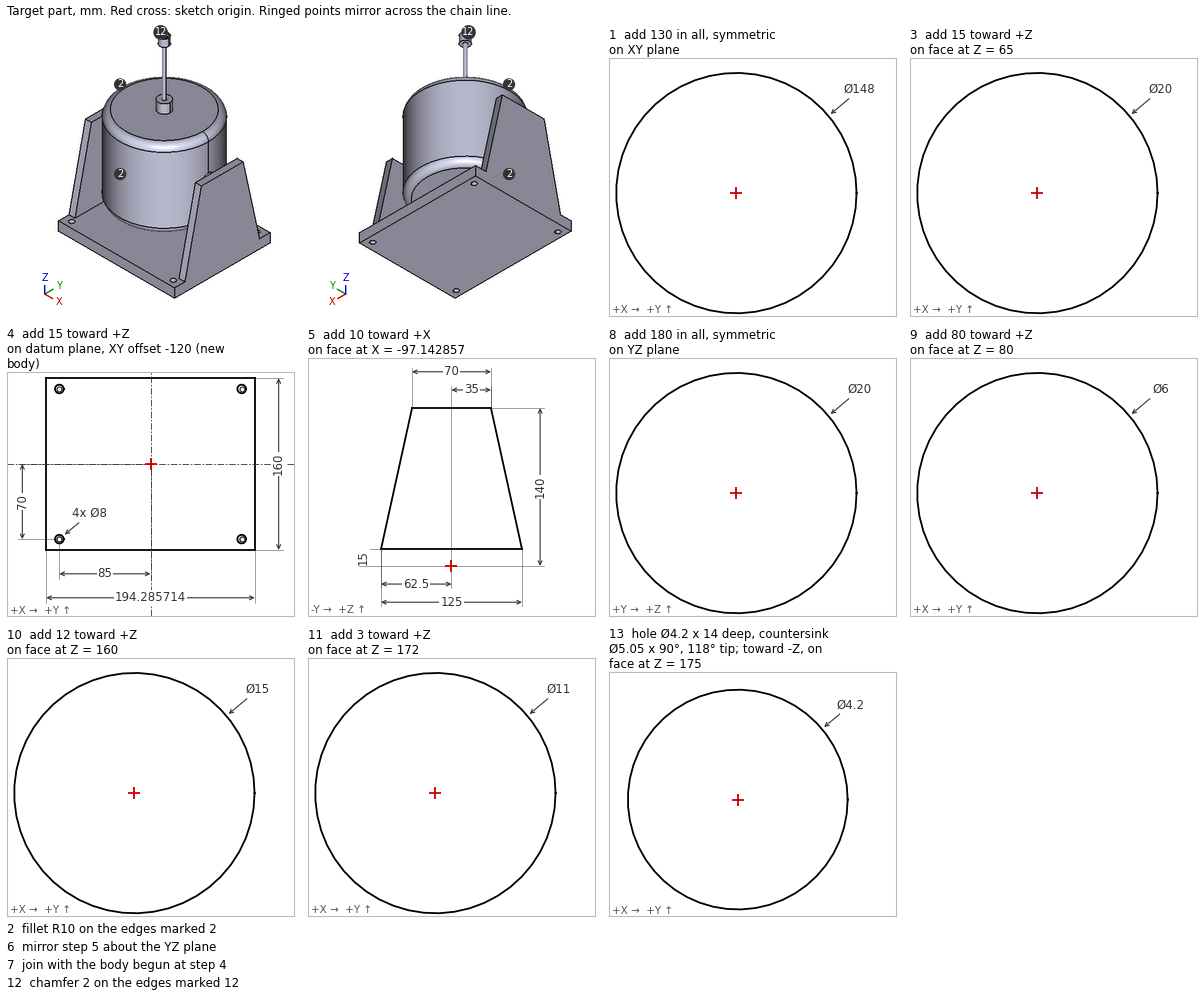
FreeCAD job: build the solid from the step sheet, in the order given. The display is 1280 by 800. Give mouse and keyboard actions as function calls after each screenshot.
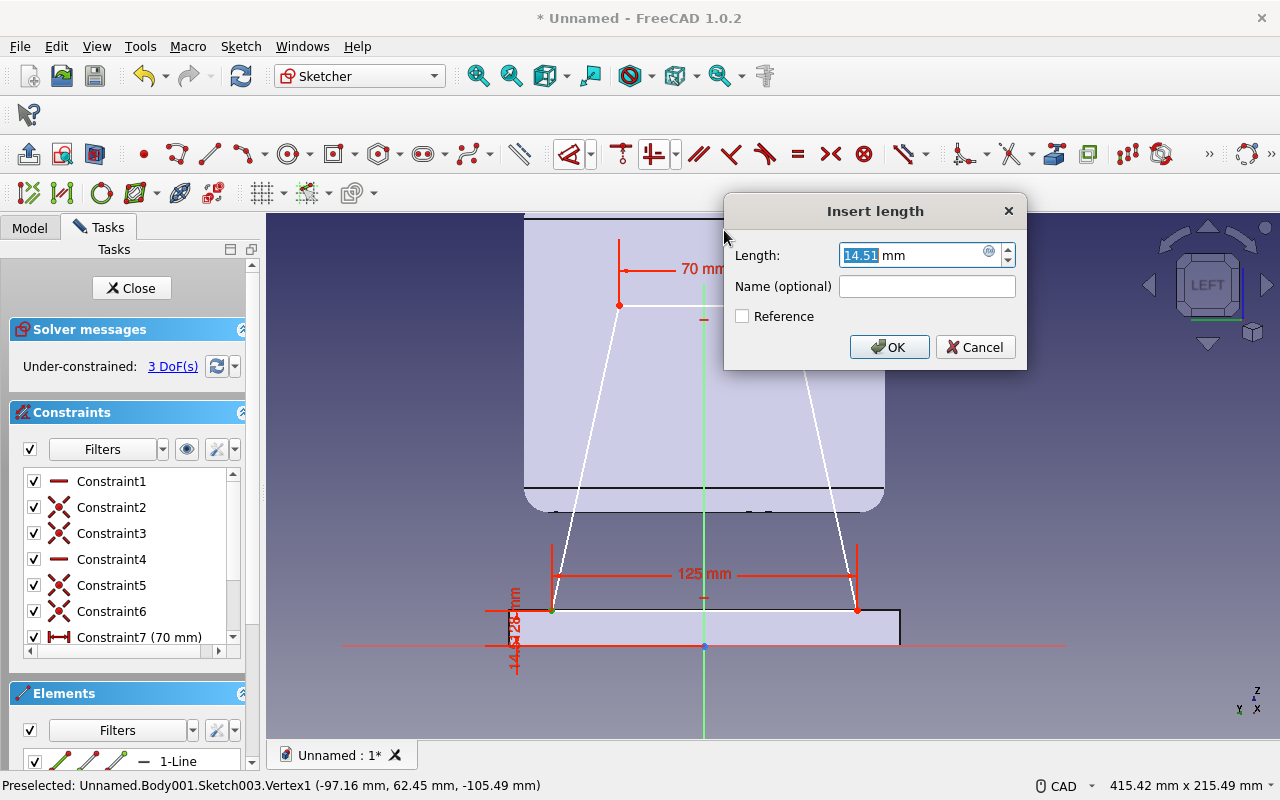
text(15)
key(Return)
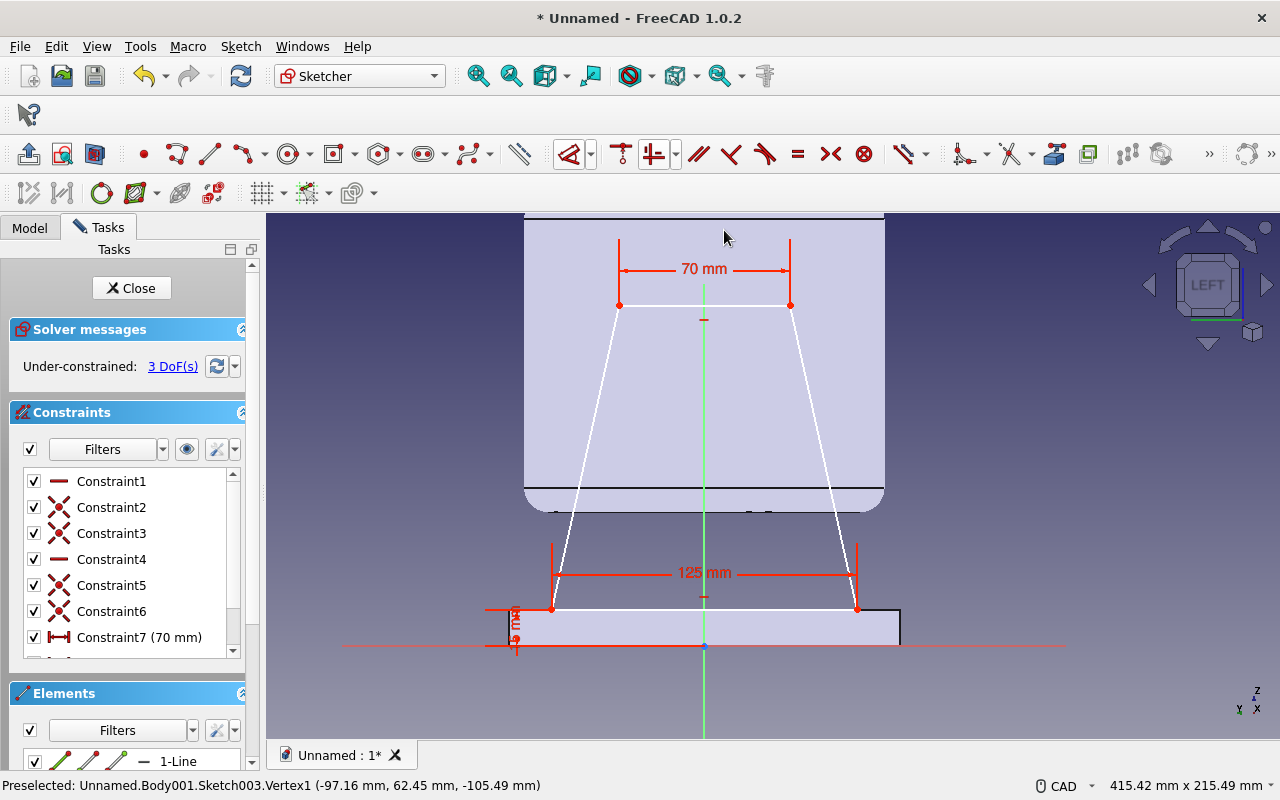
click(790, 306)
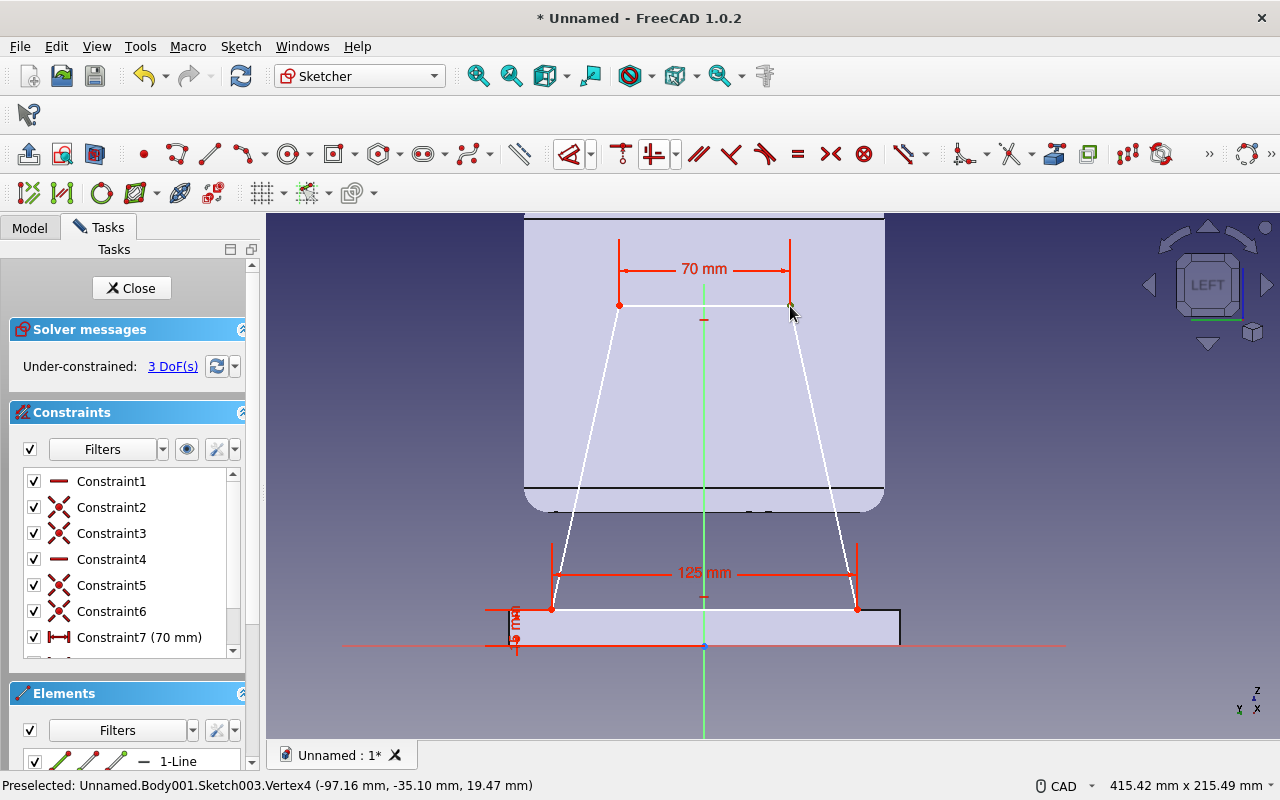
click(590, 154)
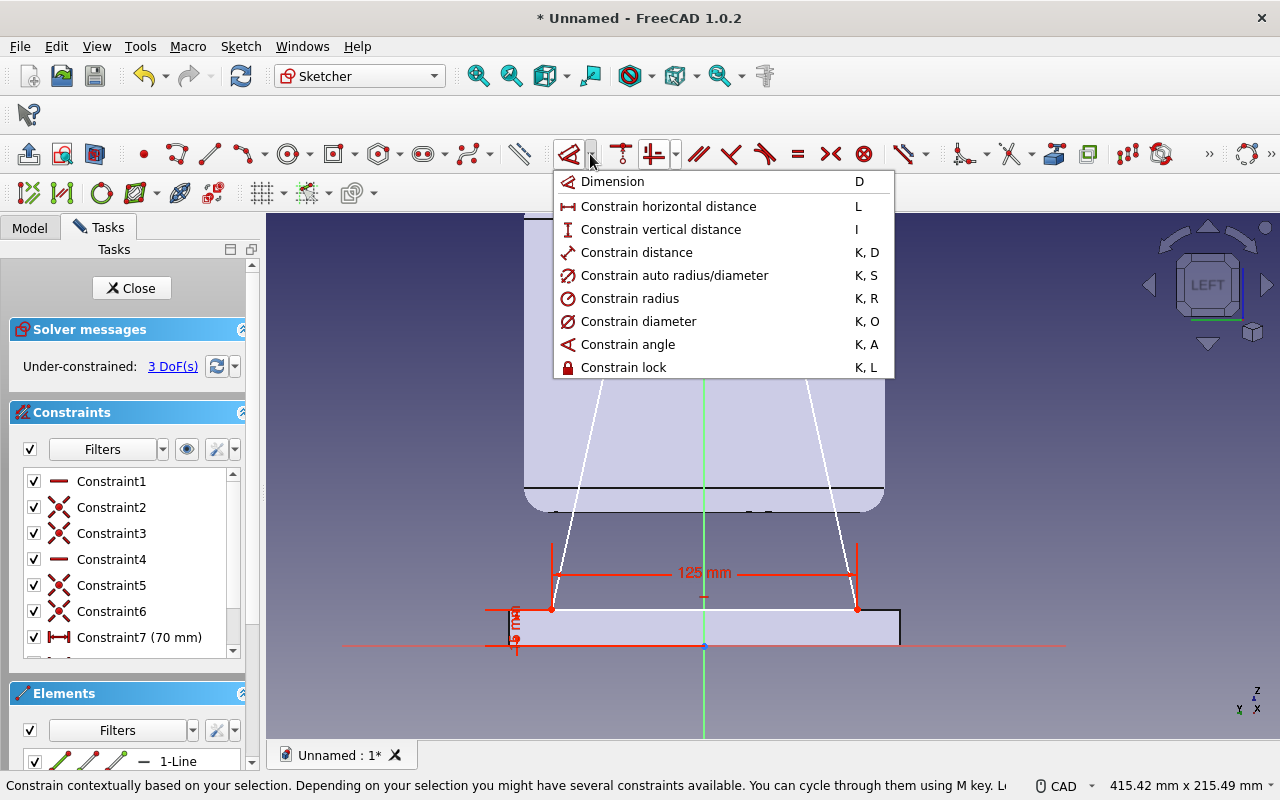
click(724, 206)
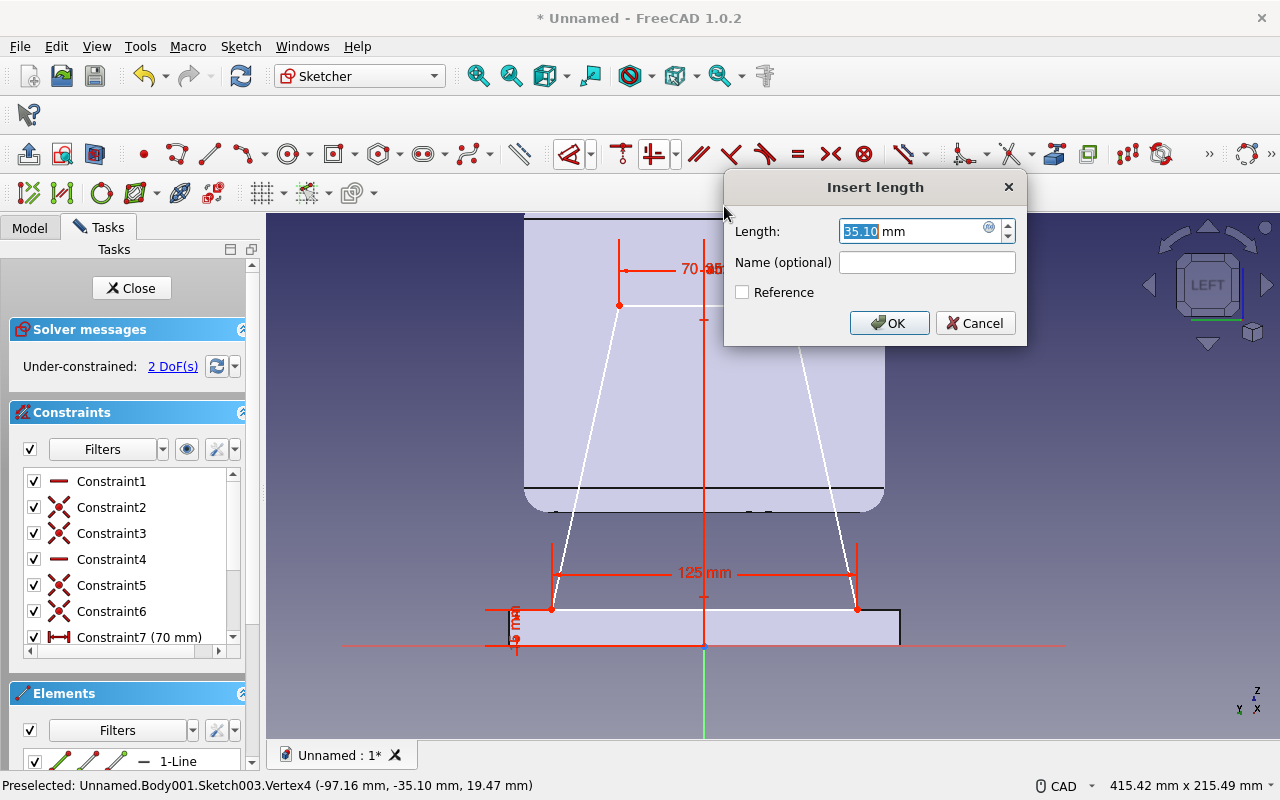
text(35)
key(Return)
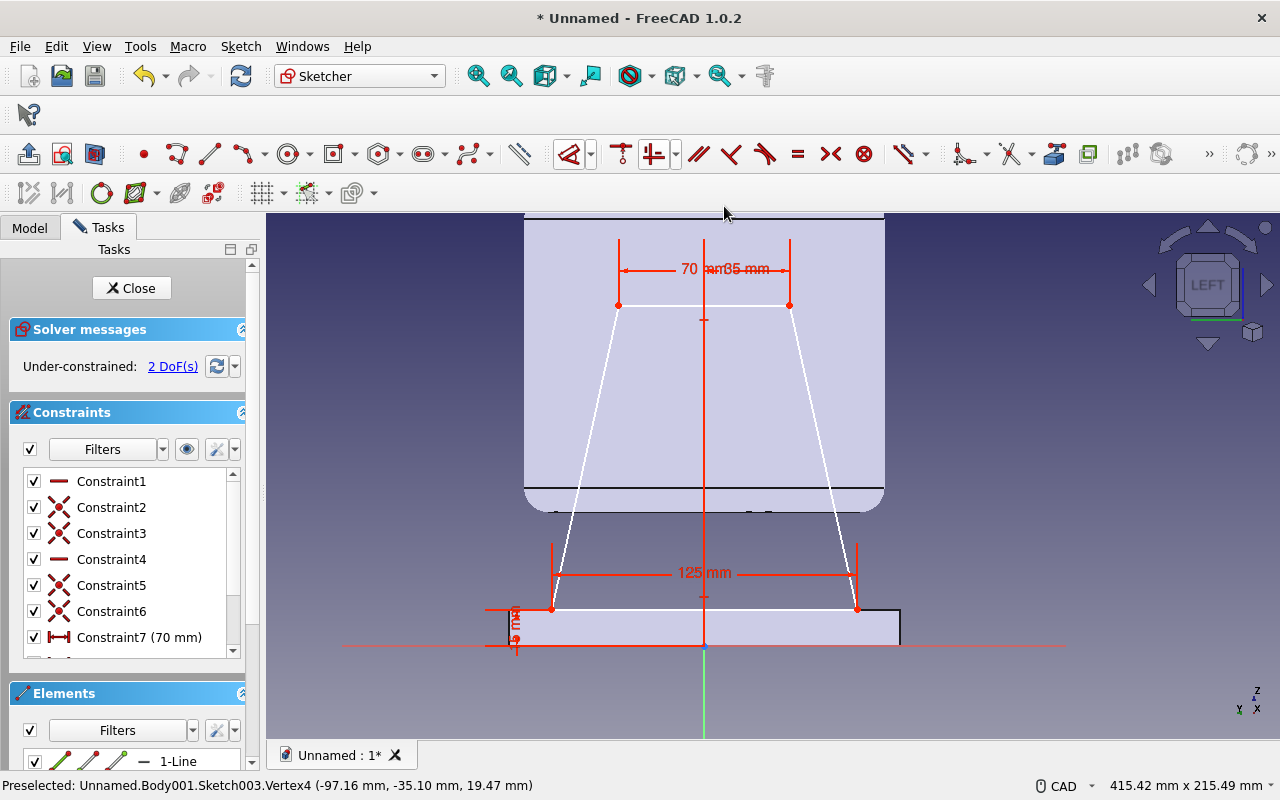
click(790, 306)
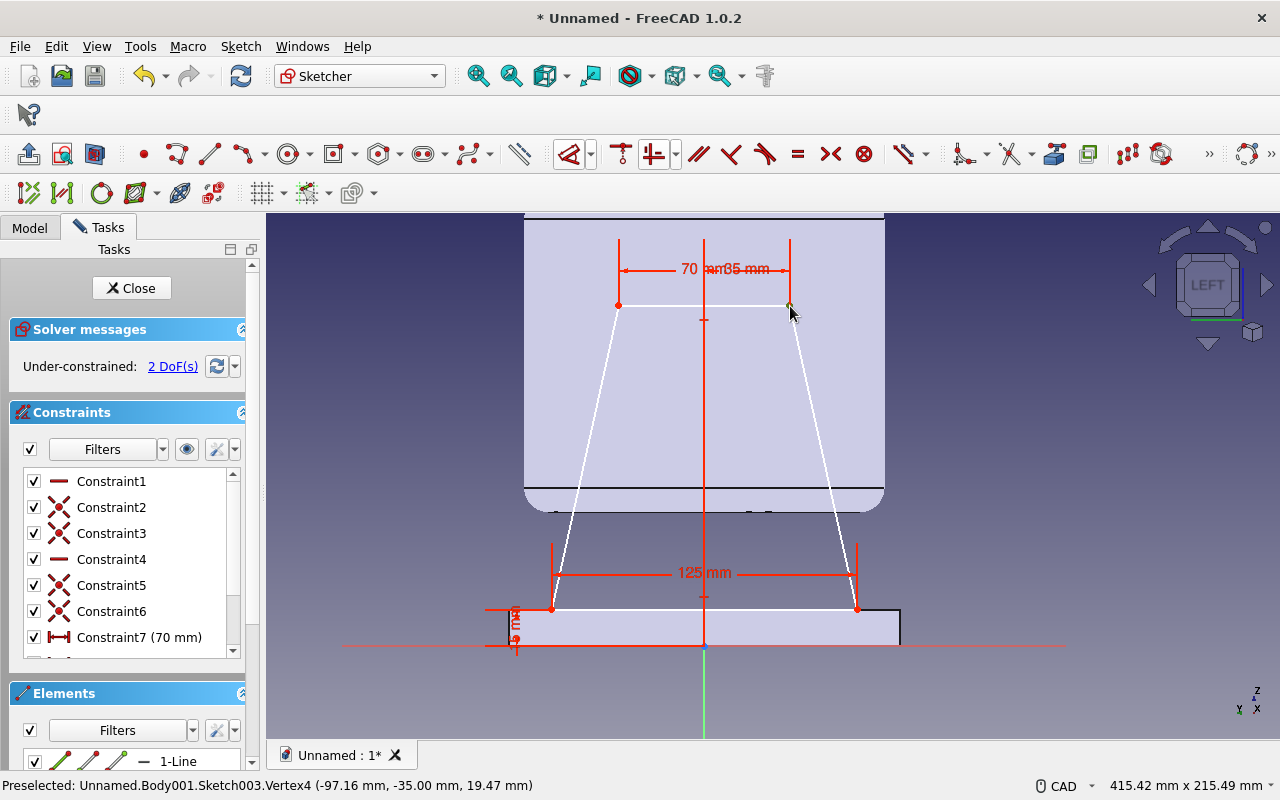
key(i)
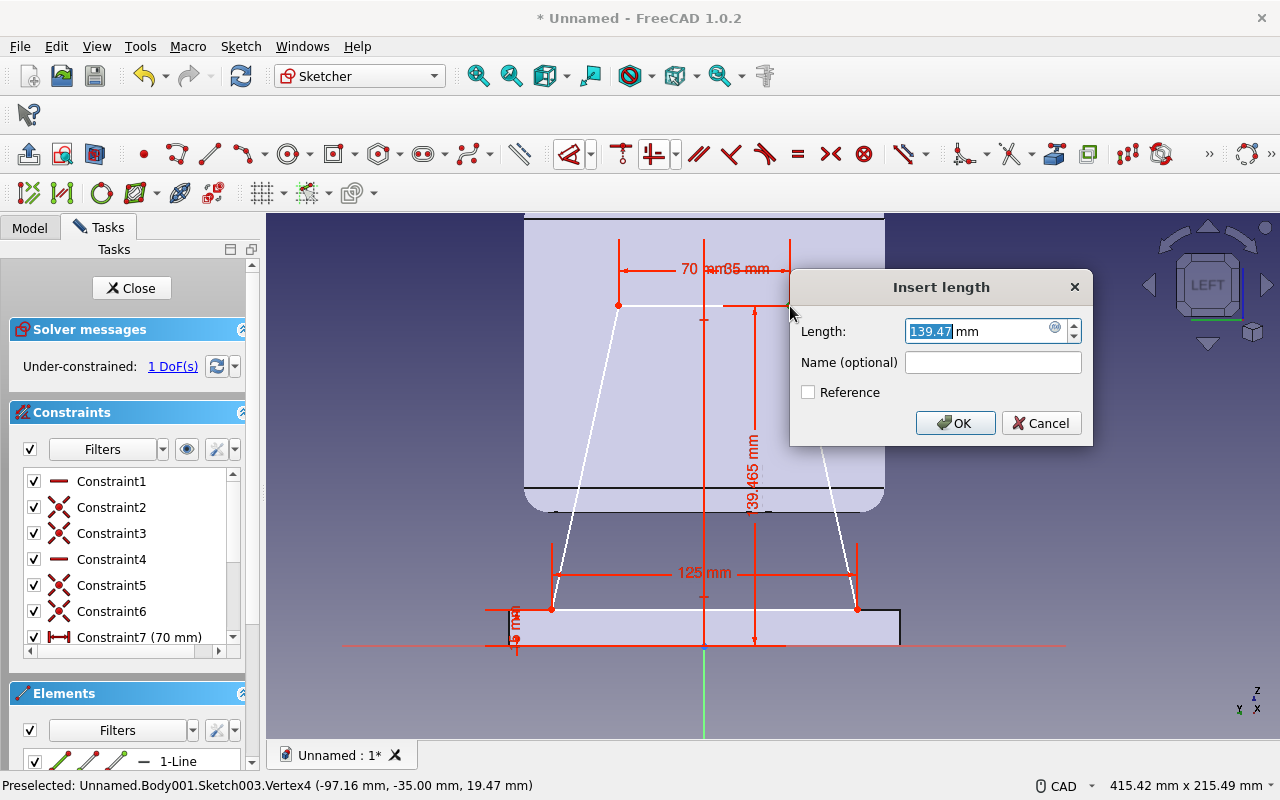
text(140)
key(Return)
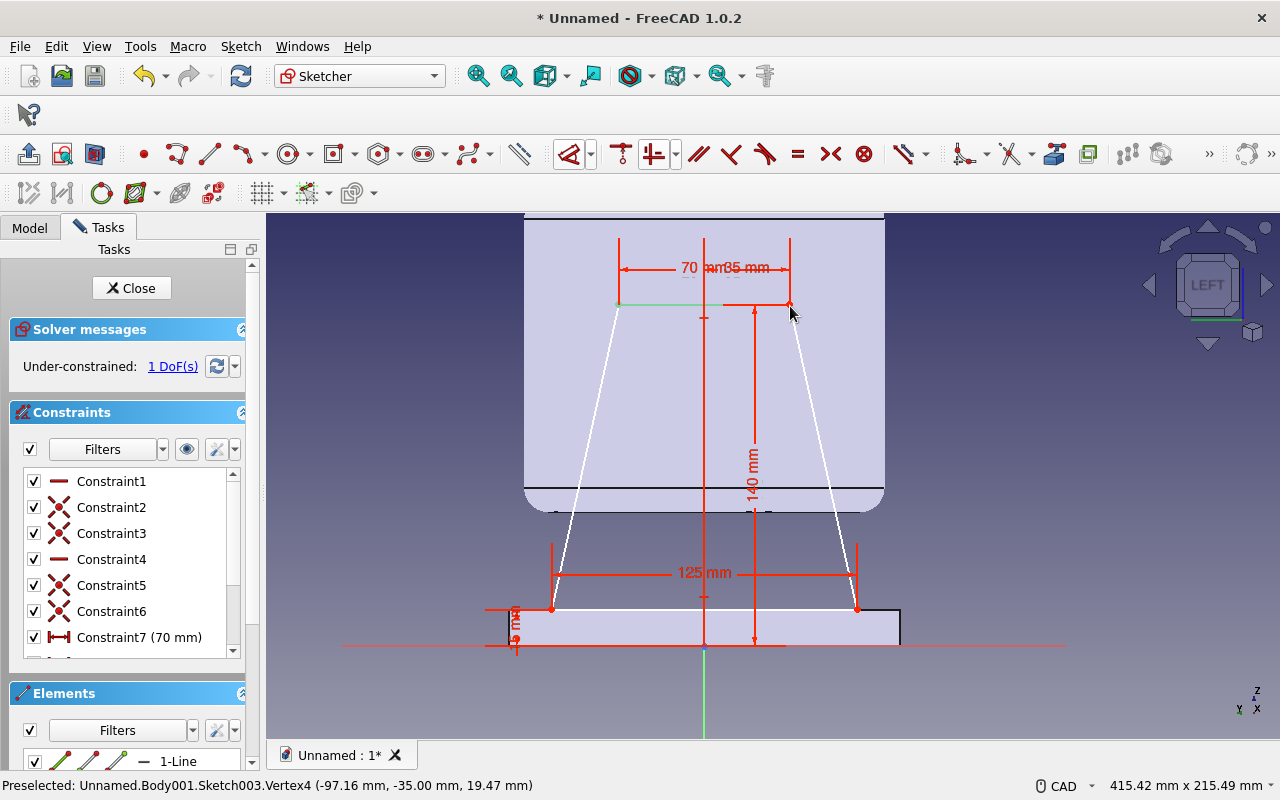
click(552, 610)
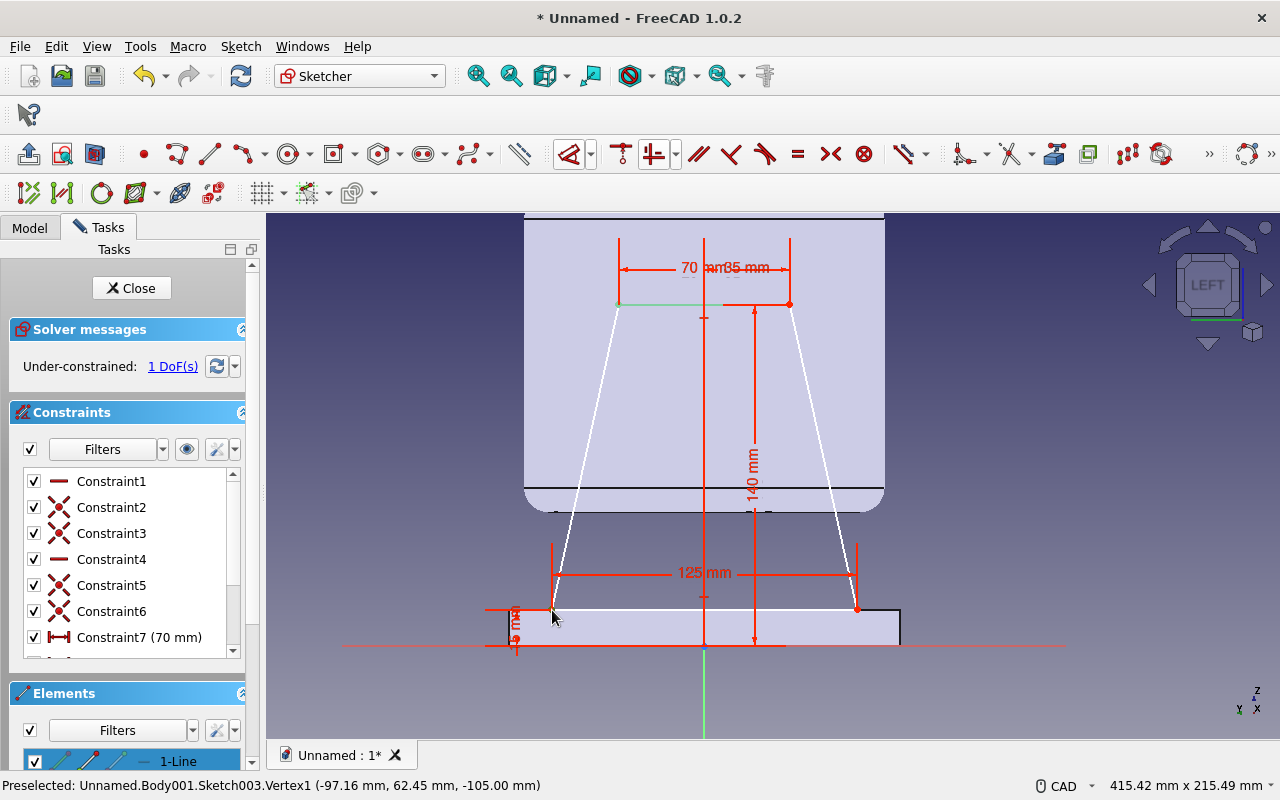
key(l)